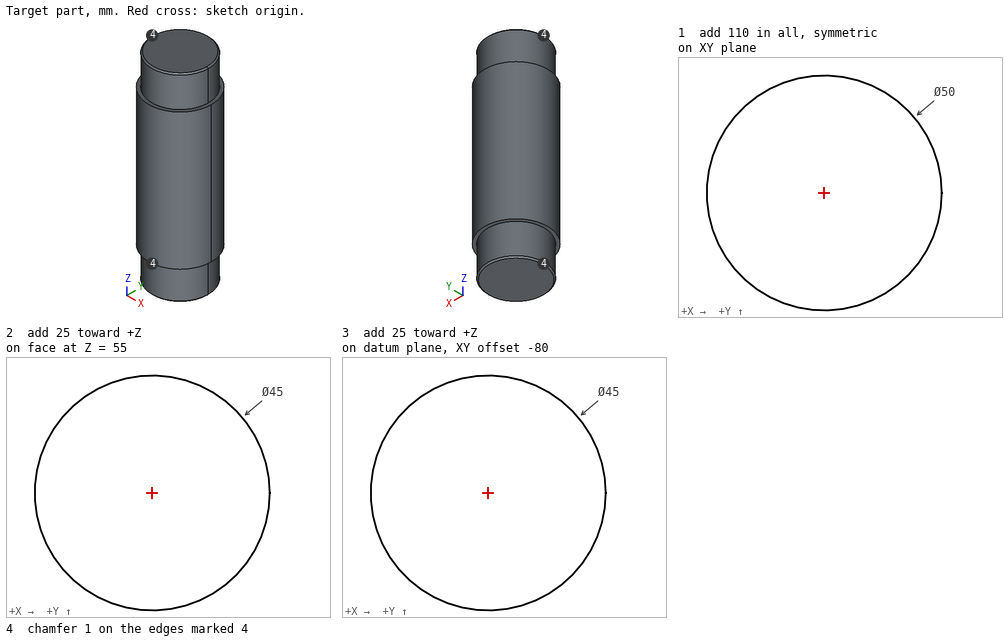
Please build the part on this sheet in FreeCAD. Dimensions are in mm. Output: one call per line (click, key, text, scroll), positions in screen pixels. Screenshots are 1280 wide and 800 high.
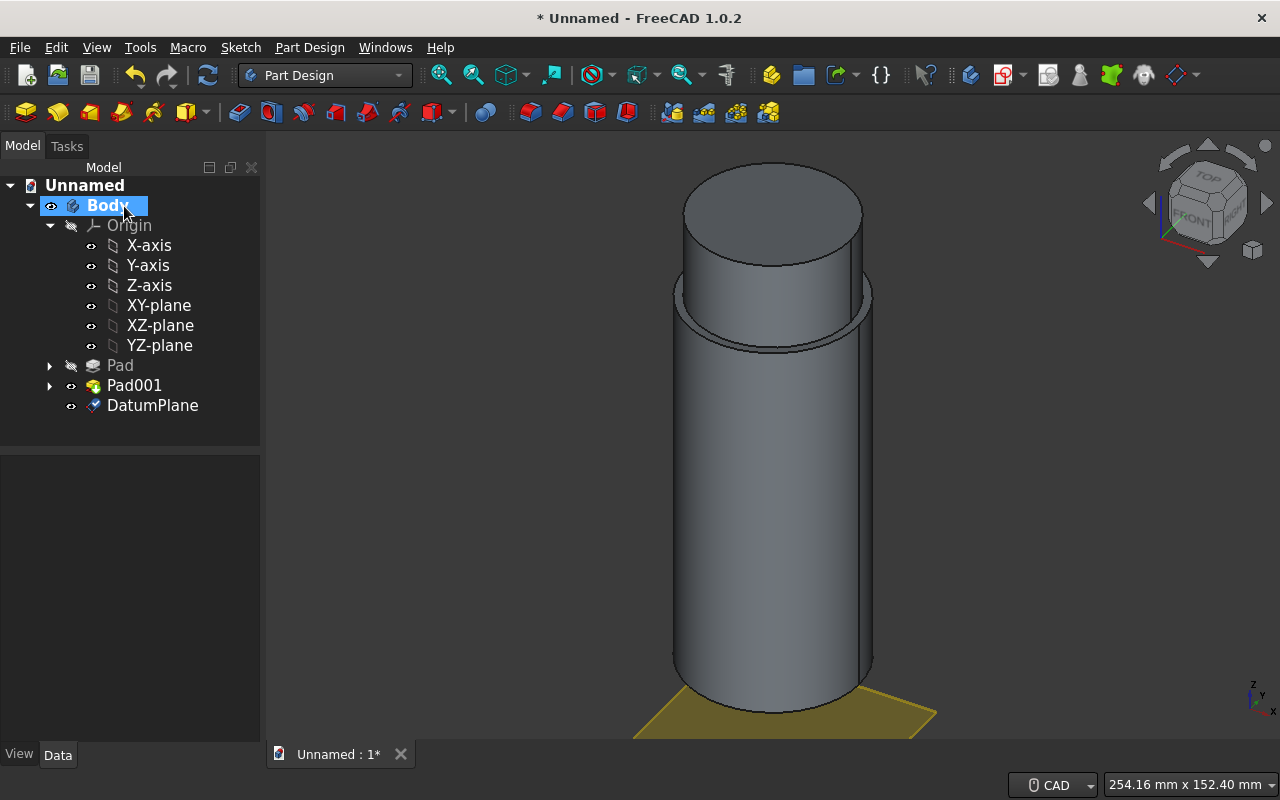
click(116, 406)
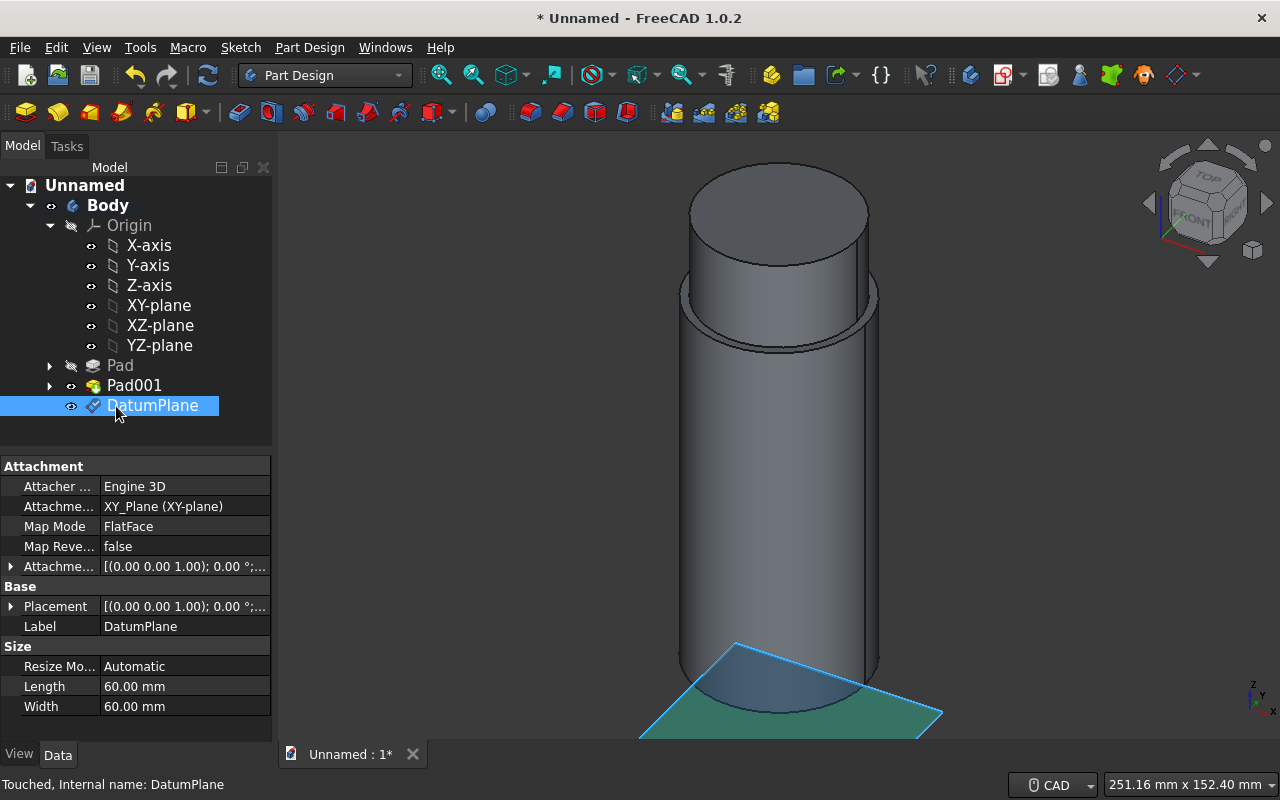
click(1004, 76)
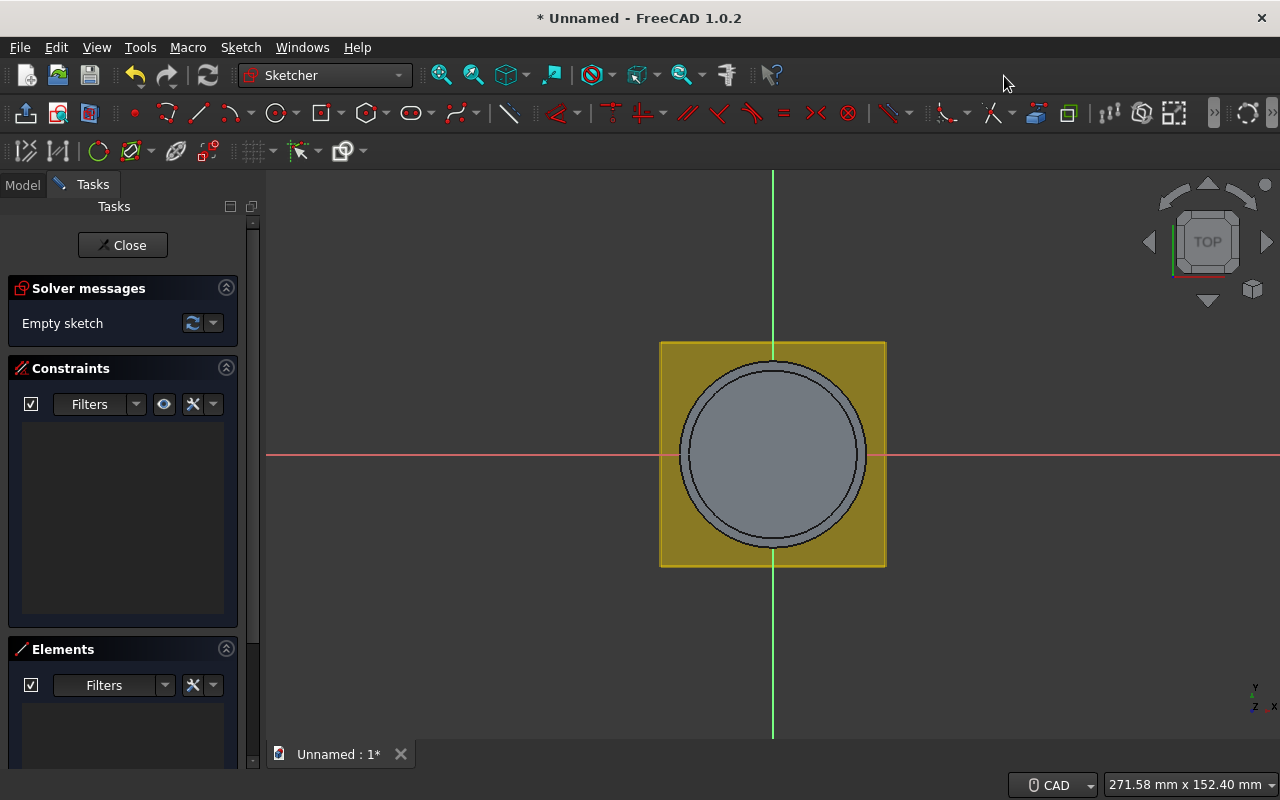
click(90, 114)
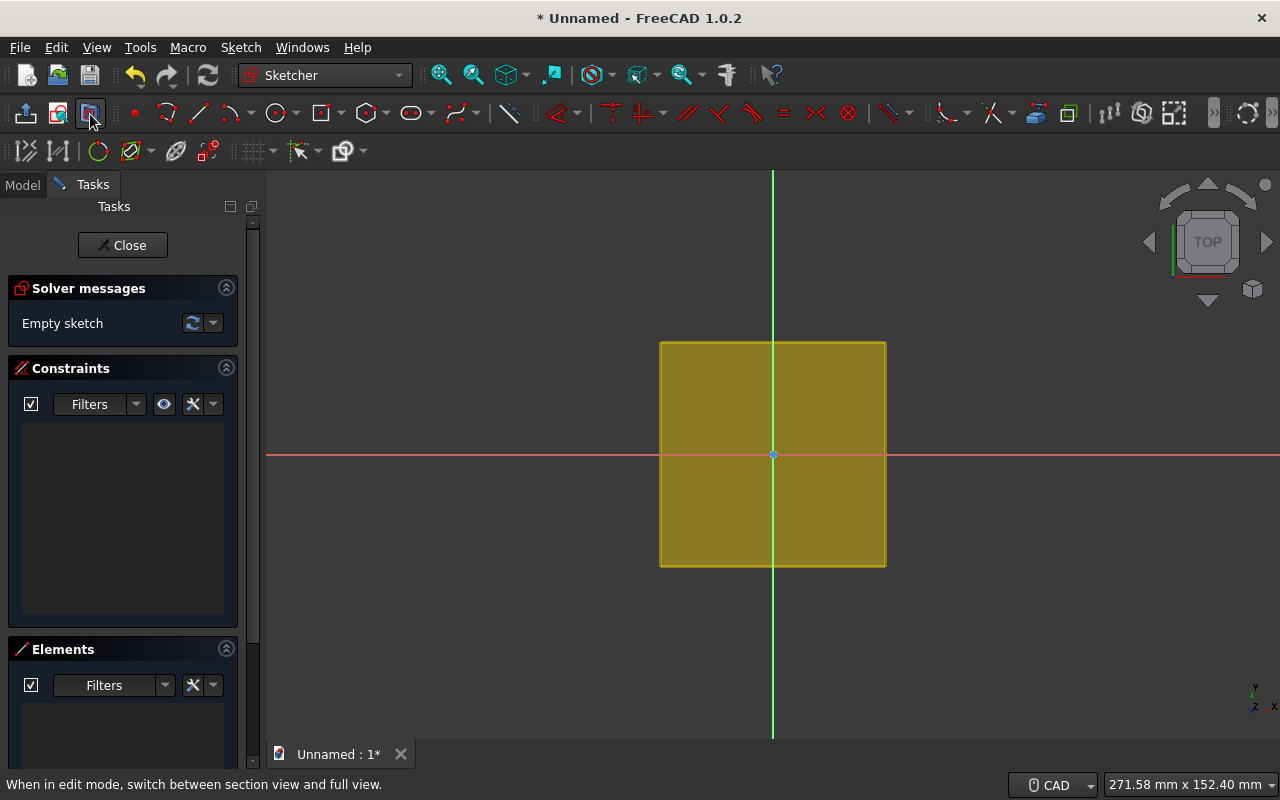
scroll(829, 455, up, 4)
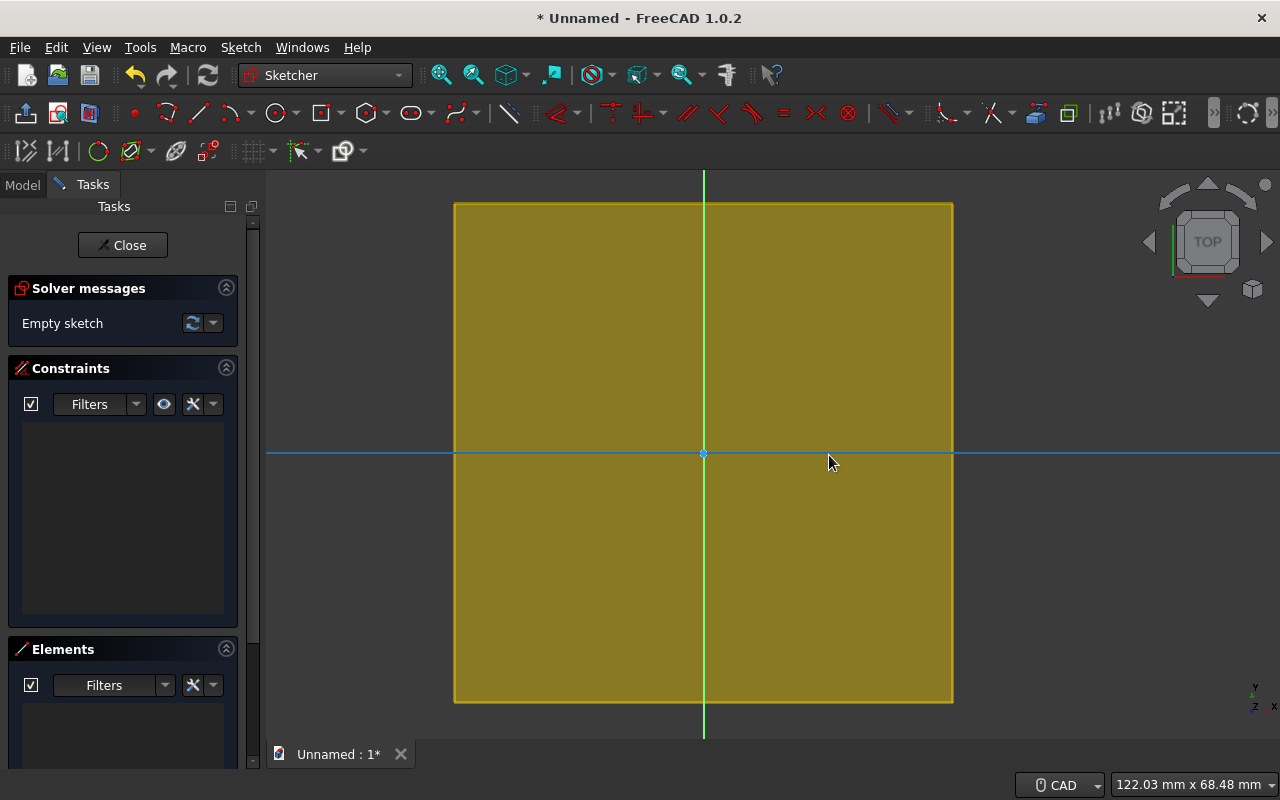
key(g)
key(c)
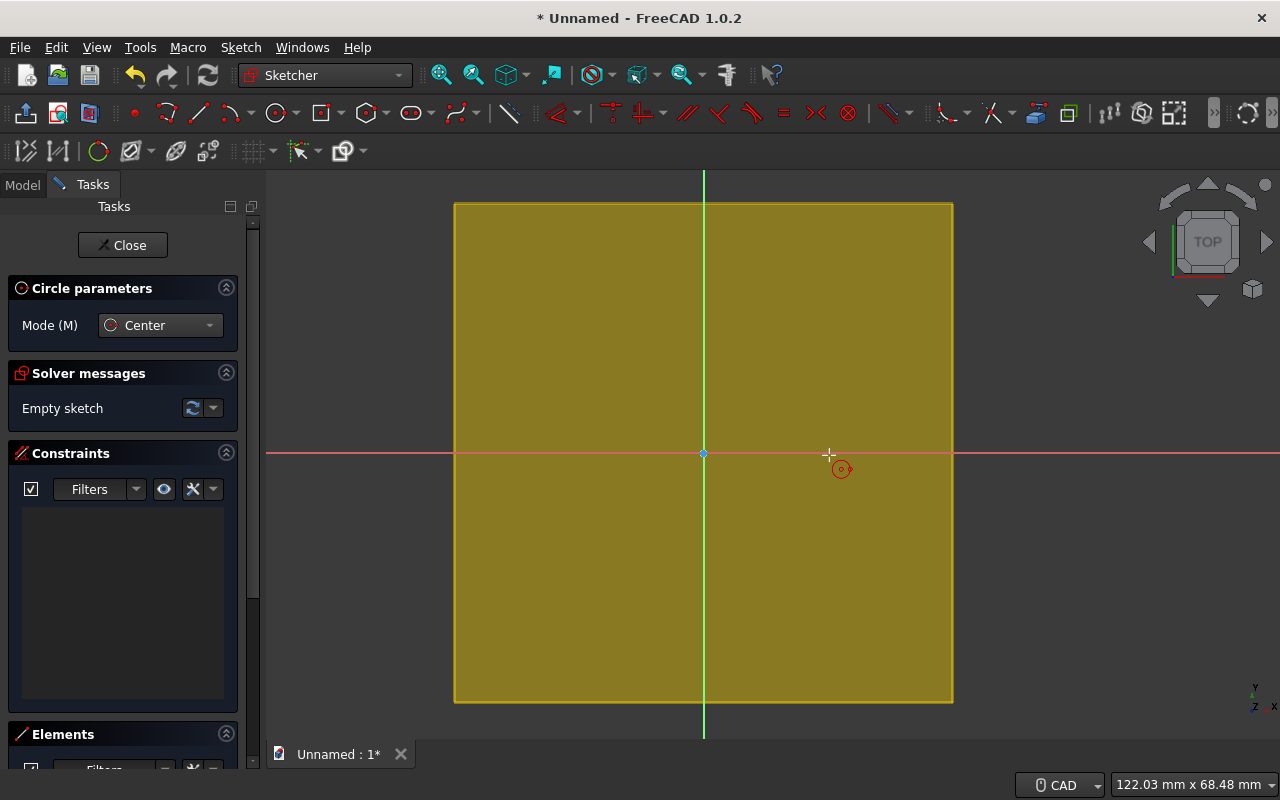
click(704, 453)
move(836, 321)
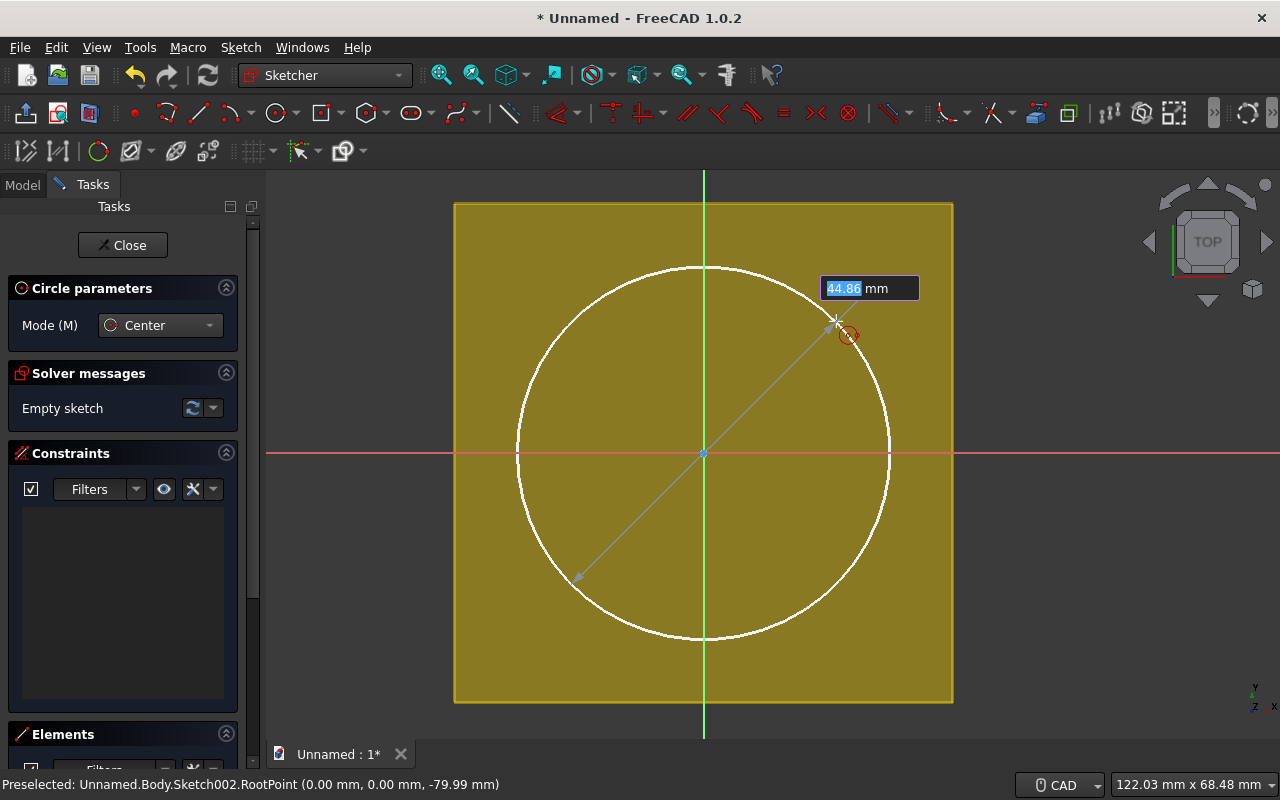
text(45)
key(Return)
key(Escape)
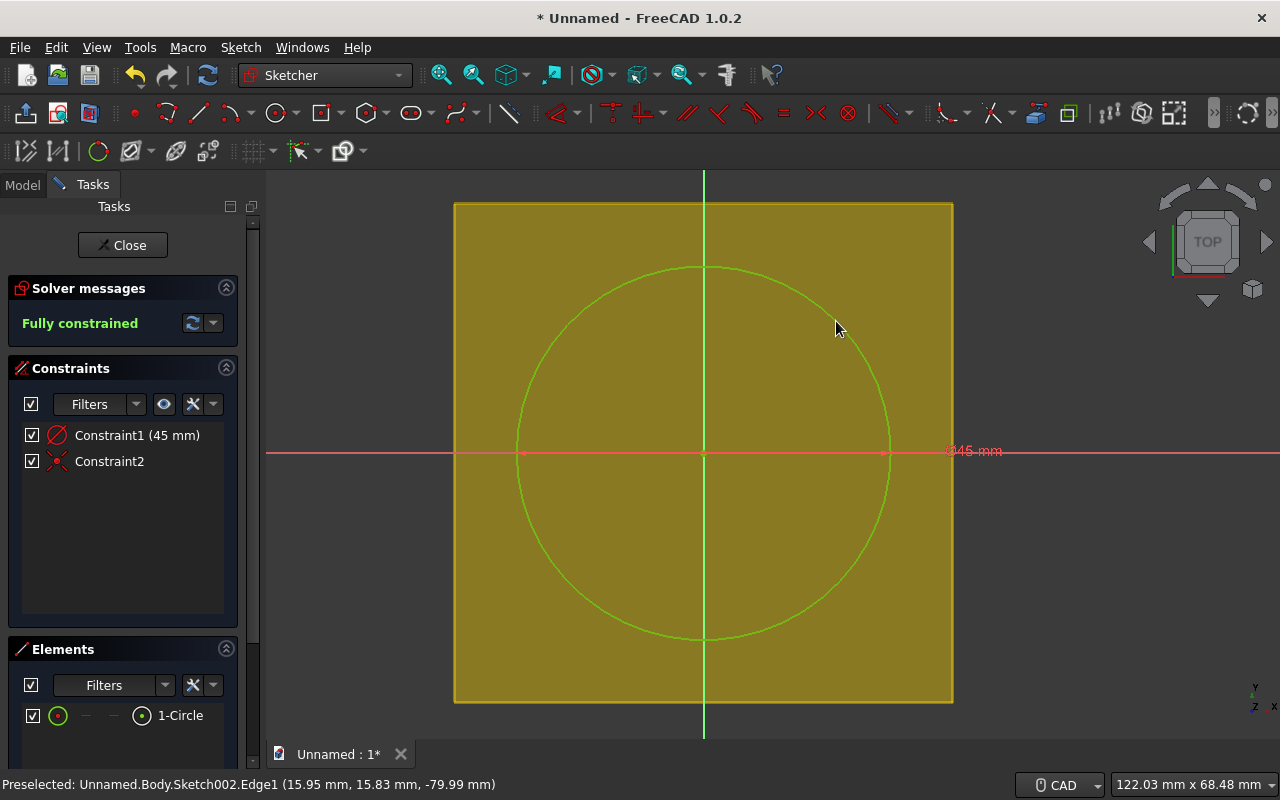
click(123, 245)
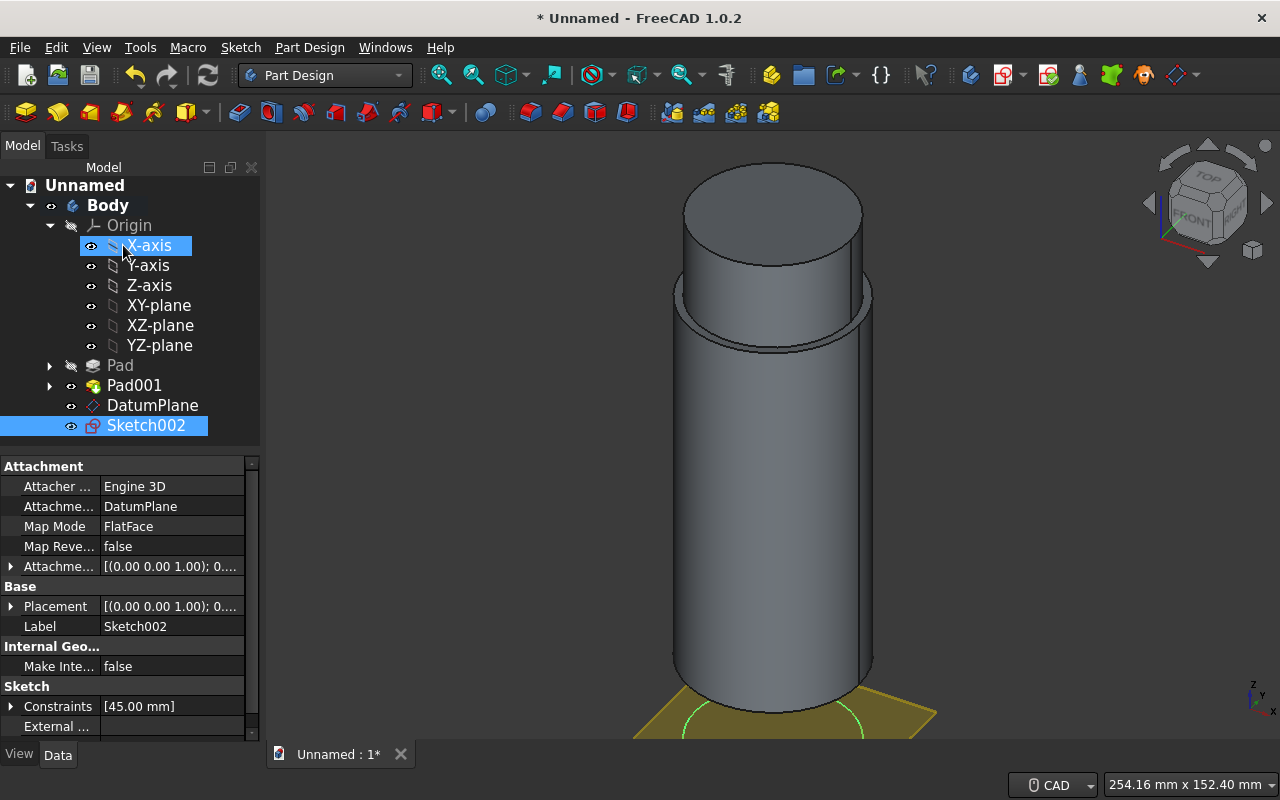
click(26, 112)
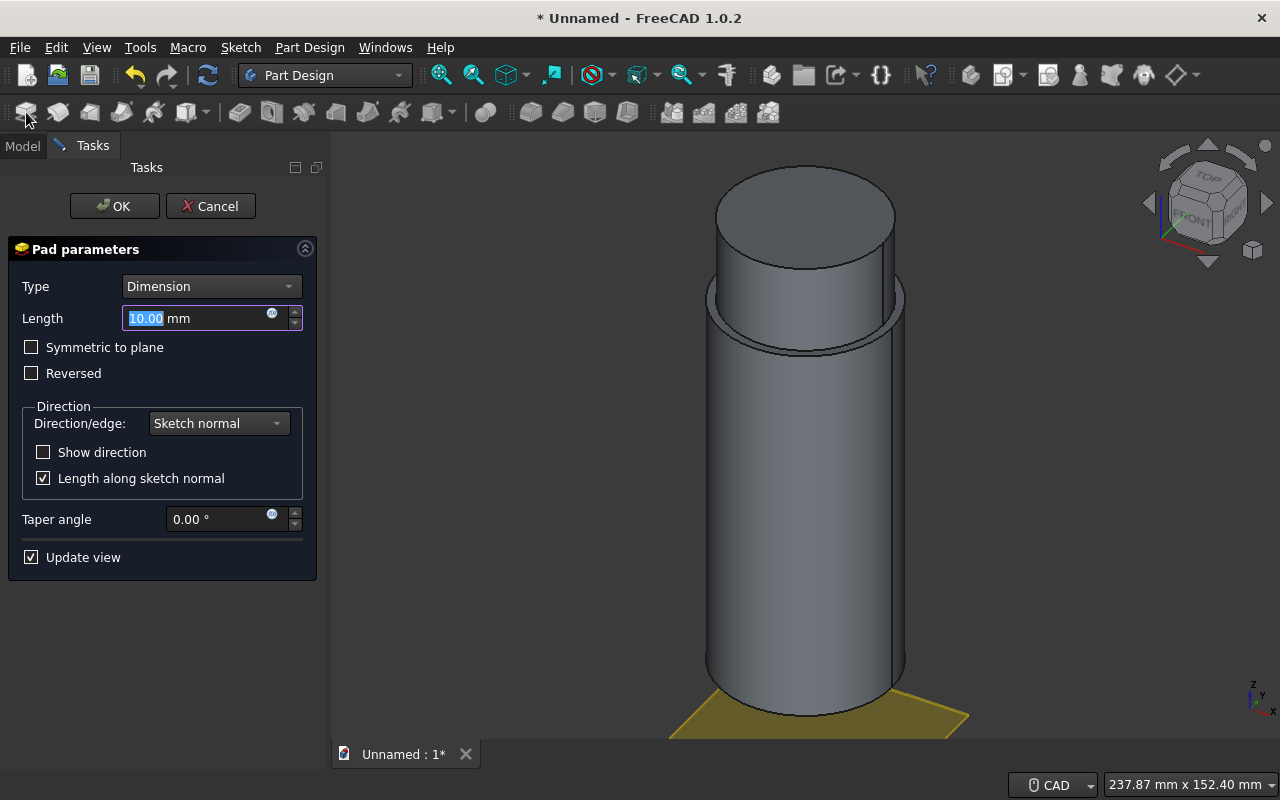
text(25)
key(Tab)